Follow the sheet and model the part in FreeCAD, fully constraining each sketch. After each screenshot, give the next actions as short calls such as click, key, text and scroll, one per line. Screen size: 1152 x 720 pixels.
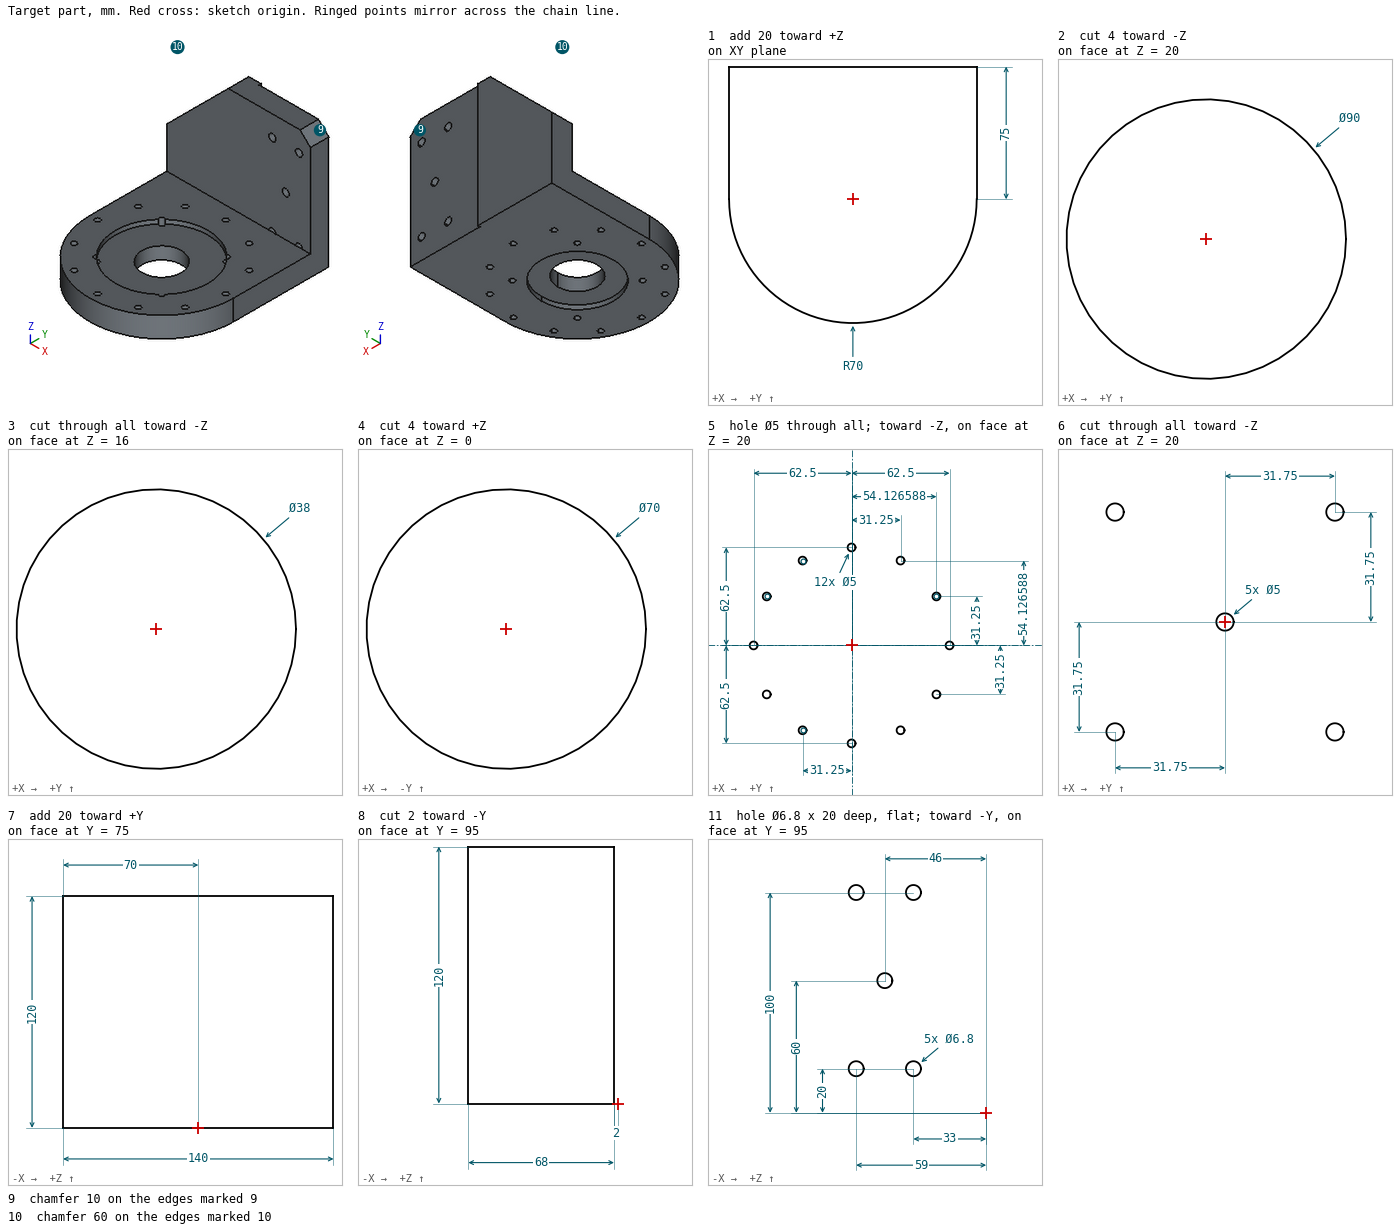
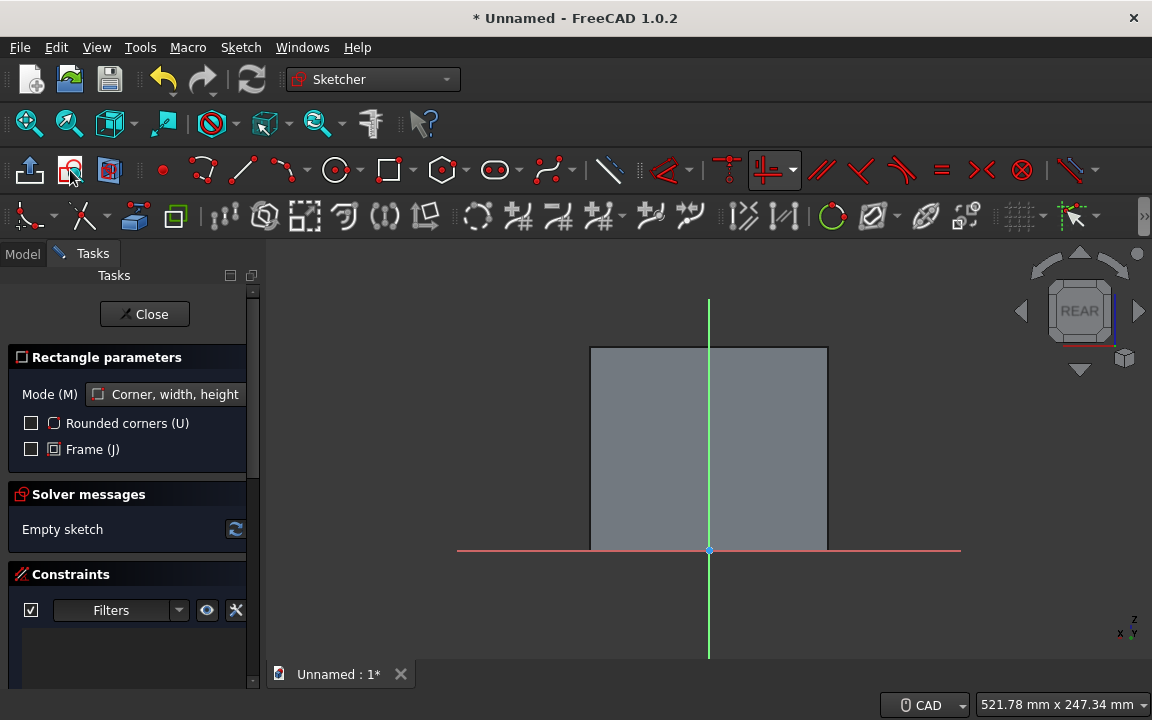
click(590, 347)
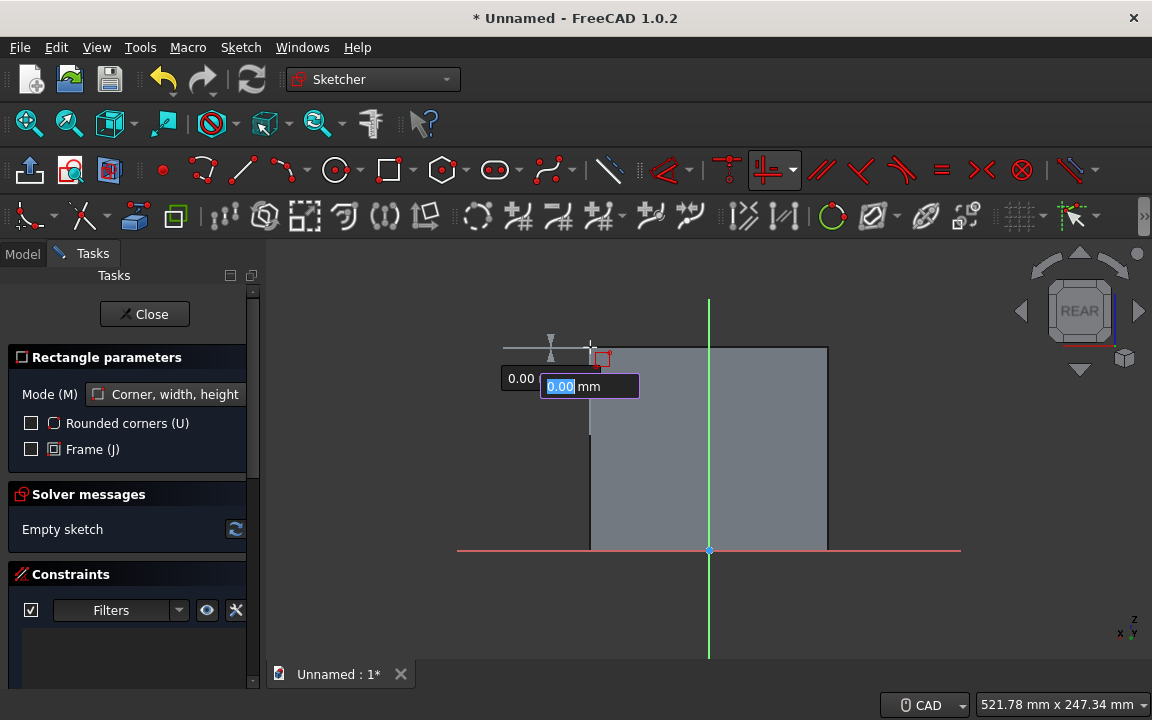
scroll(706, 551, up, 8)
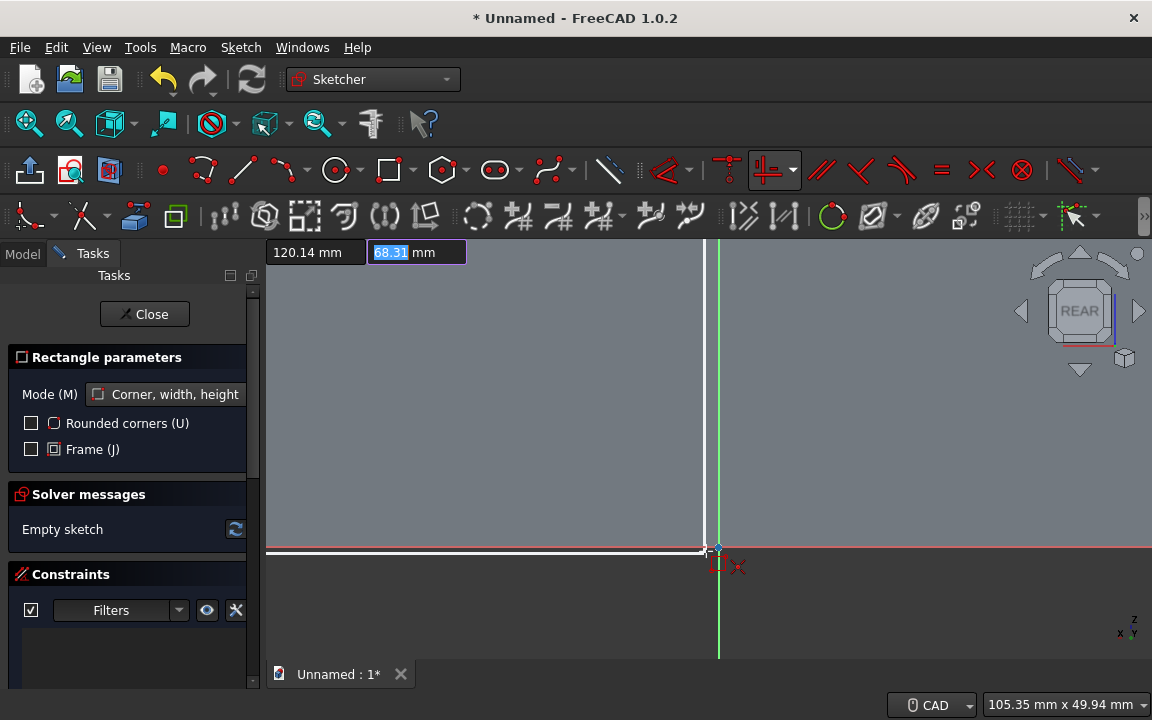
click(702, 547)
key(Escape)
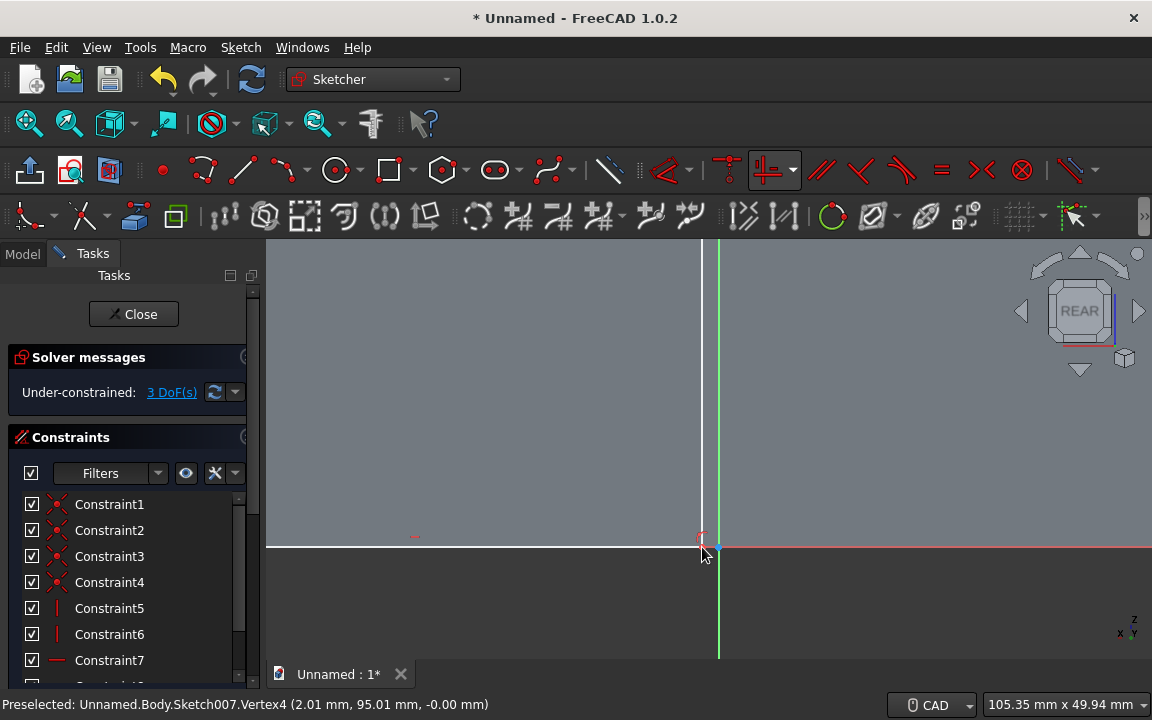
key(d)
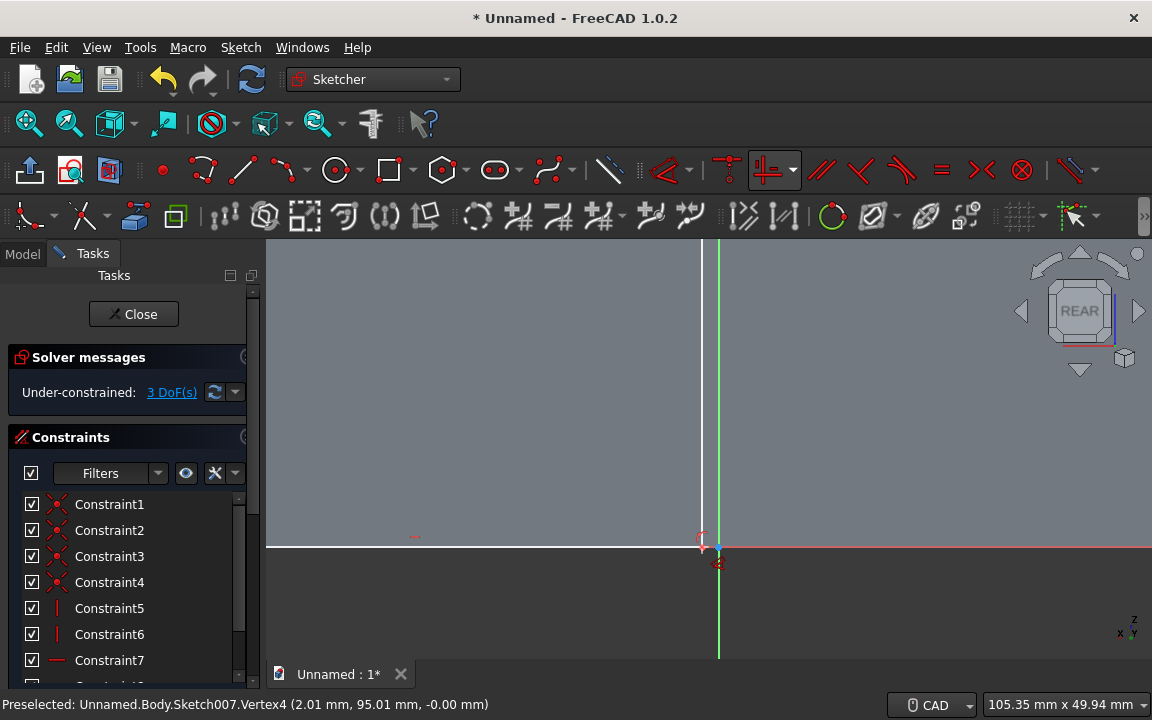
scroll(711, 582, down, 7)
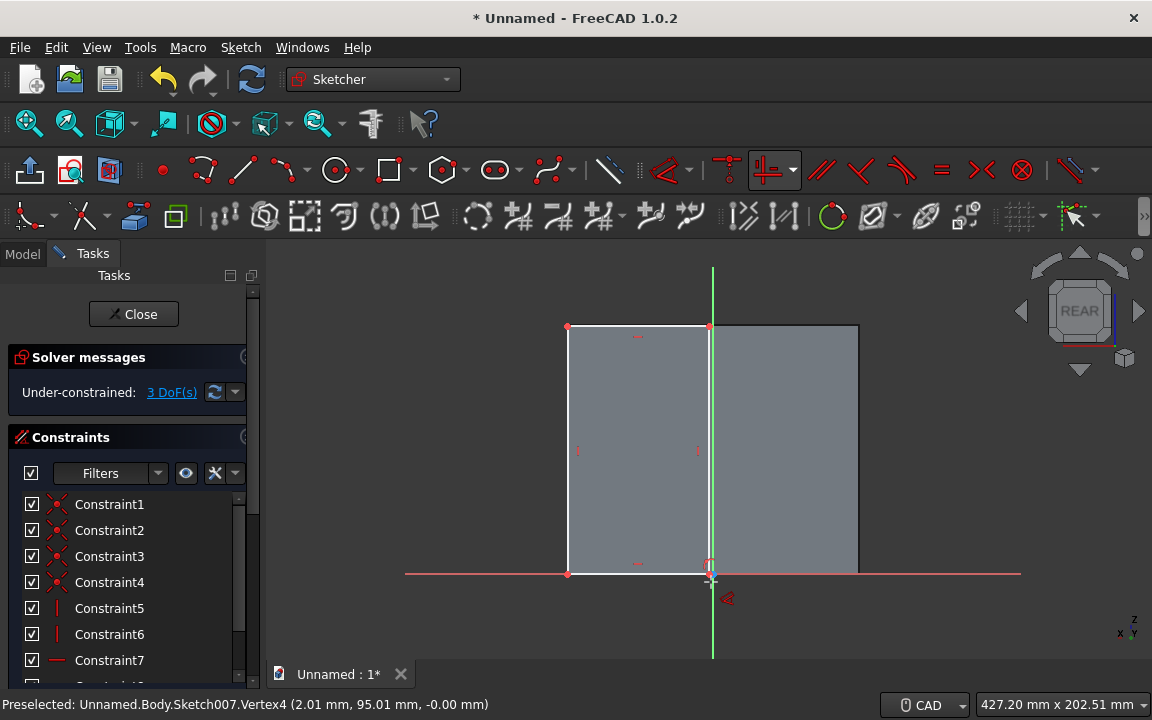
click(610, 574)
click(639, 608)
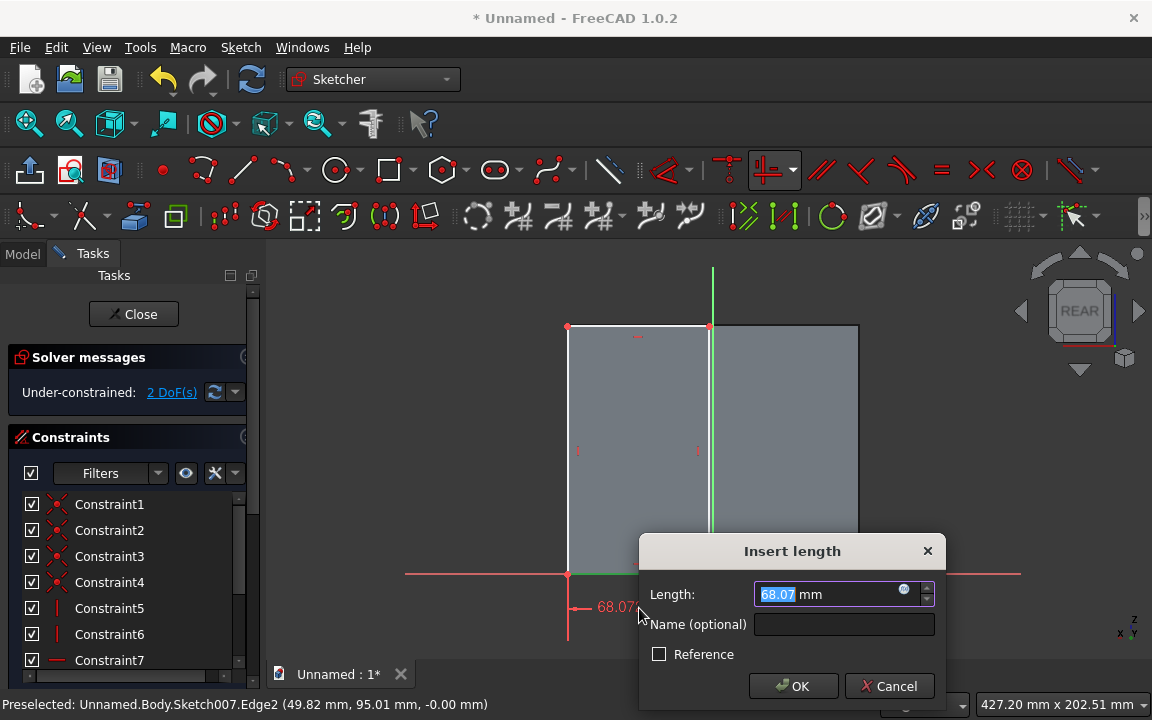
text(68)
key(Return)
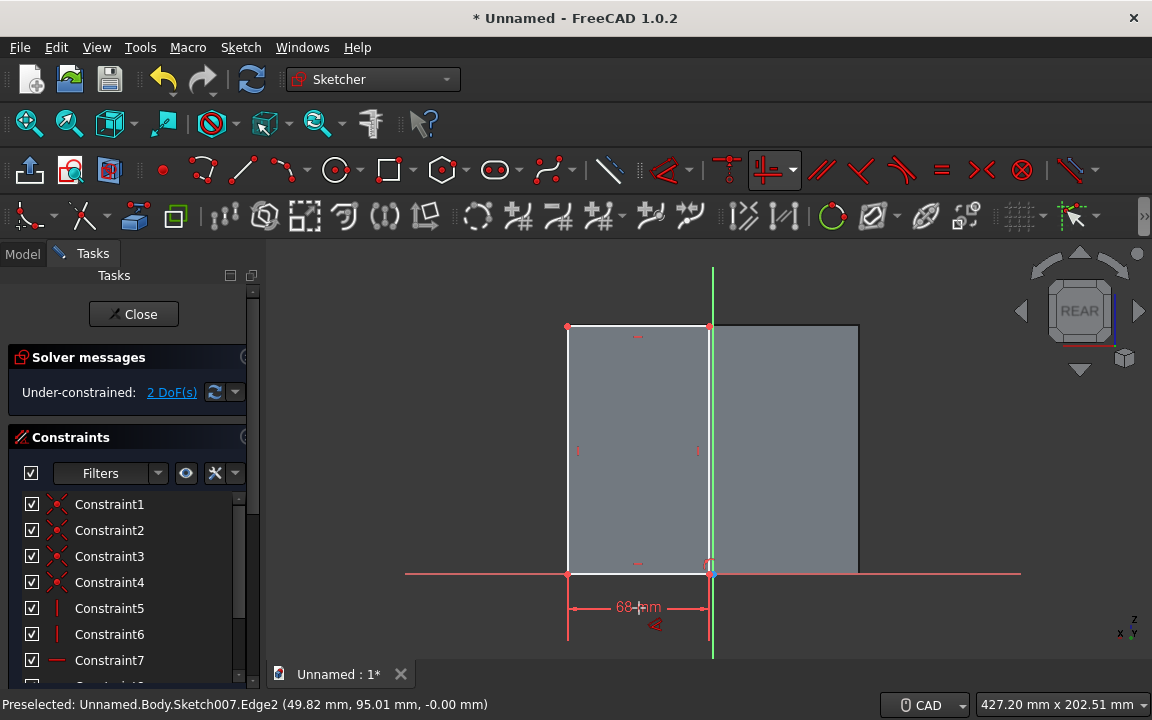
scroll(709, 574, up, 12)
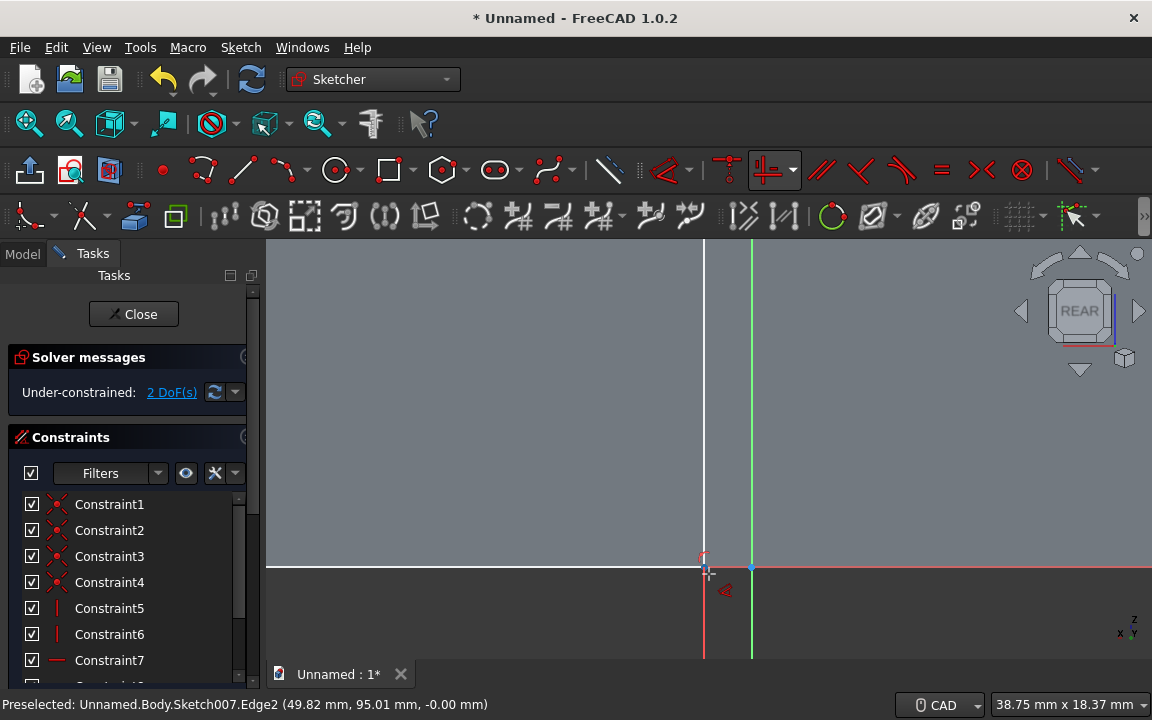
click(704, 567)
click(728, 601)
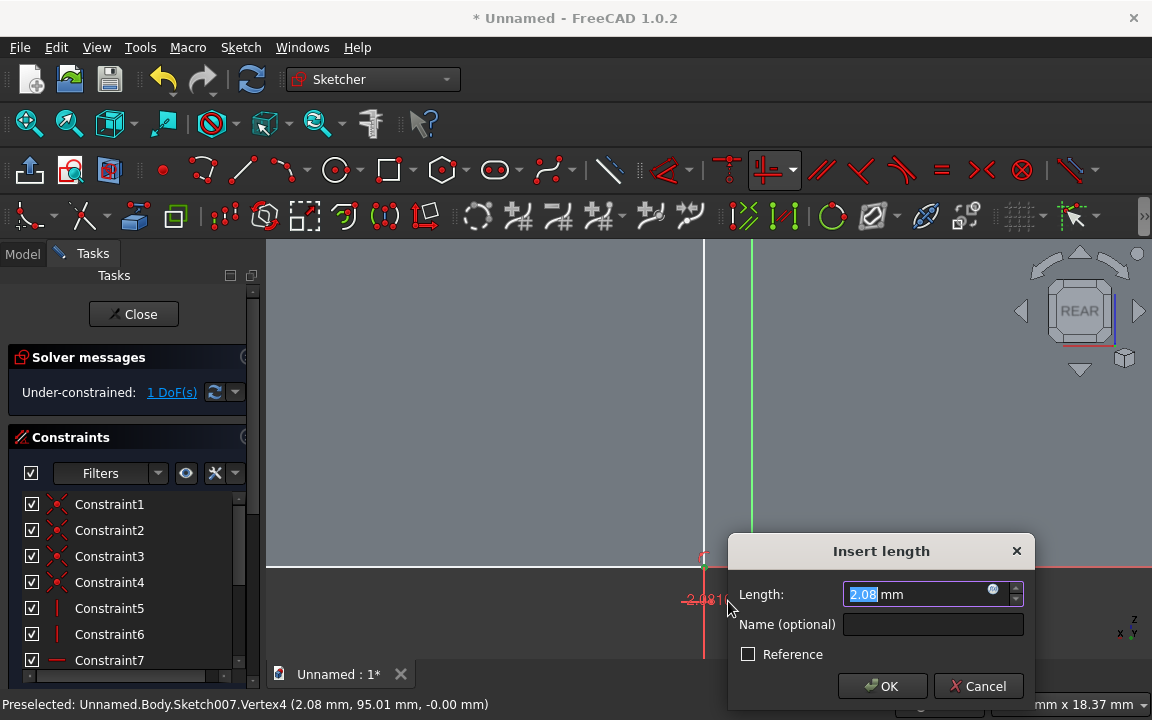
text(2)
key(Return)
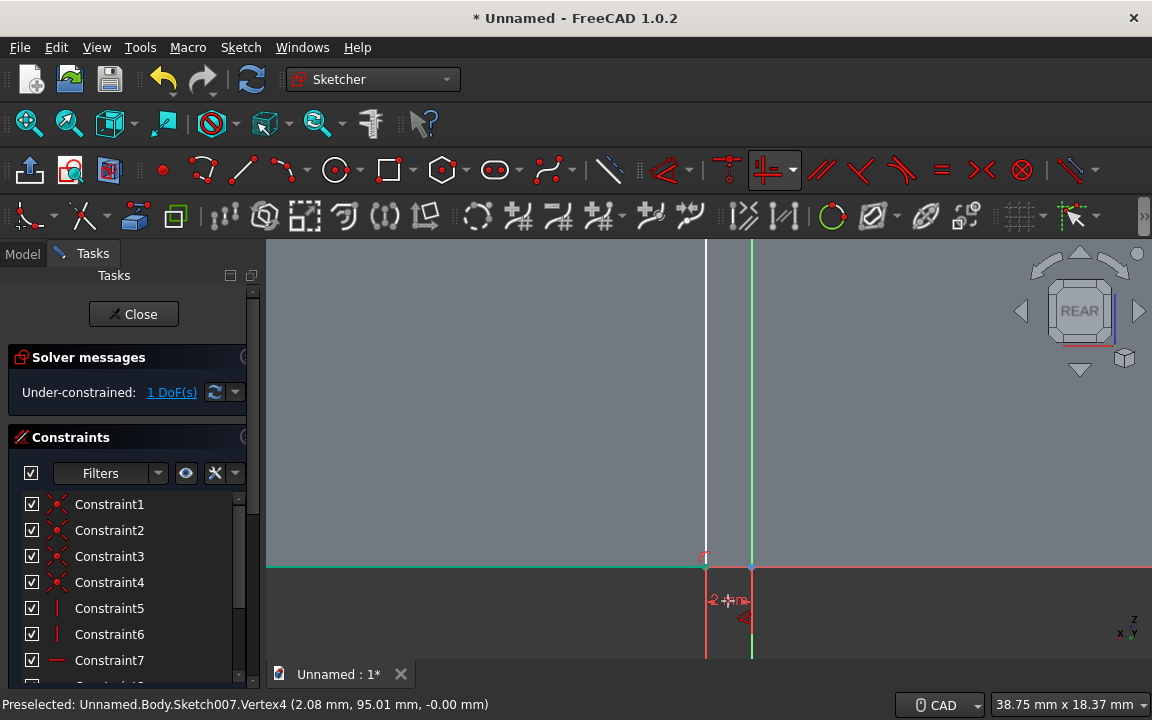
scroll(709, 574, down, 12)